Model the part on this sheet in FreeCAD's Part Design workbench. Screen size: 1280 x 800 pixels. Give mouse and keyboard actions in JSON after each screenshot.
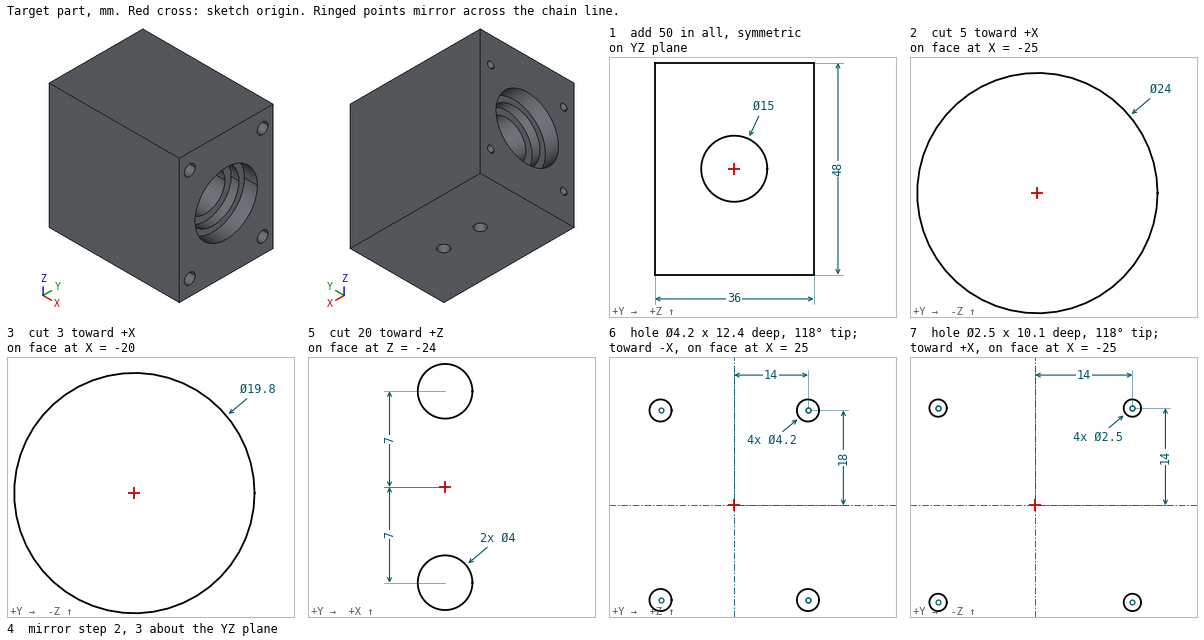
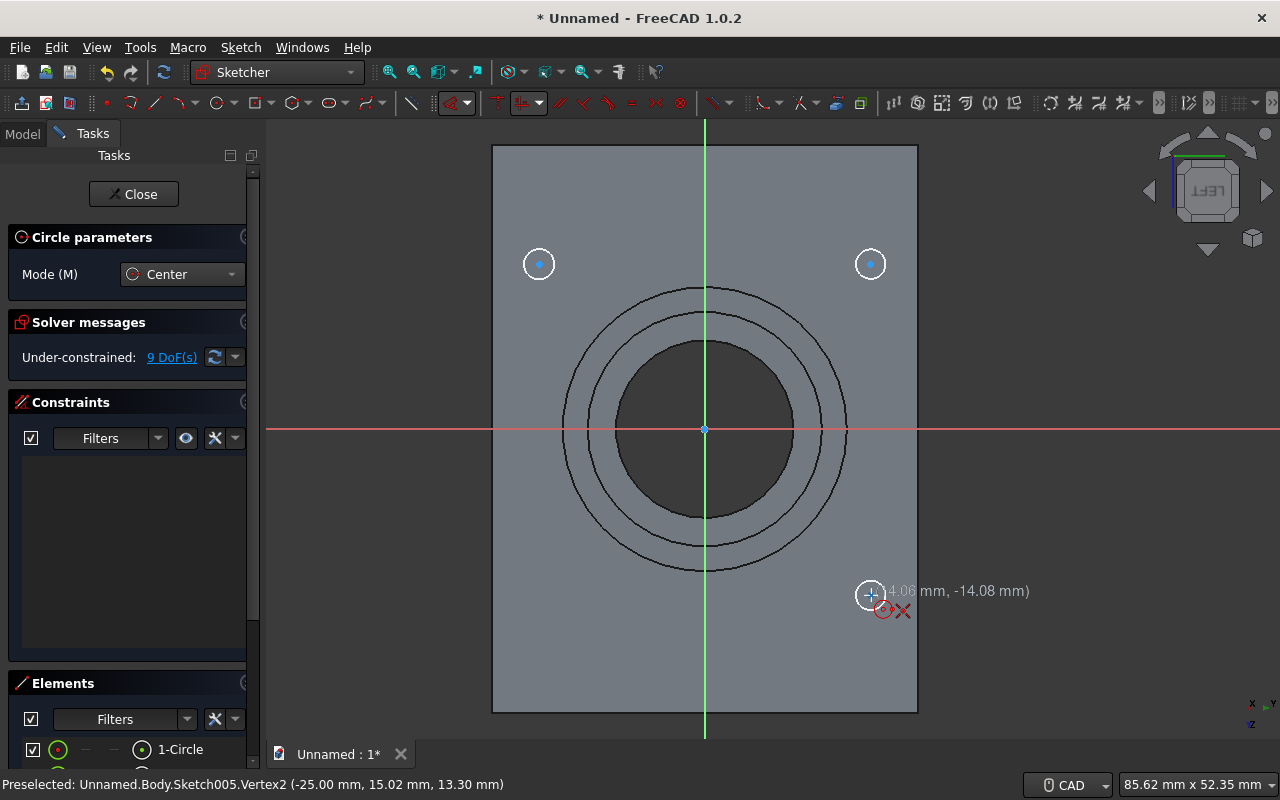
{"action": "scroll", "coordinate": [539, 595], "scroll_direction": "up", "scroll_amount": 3}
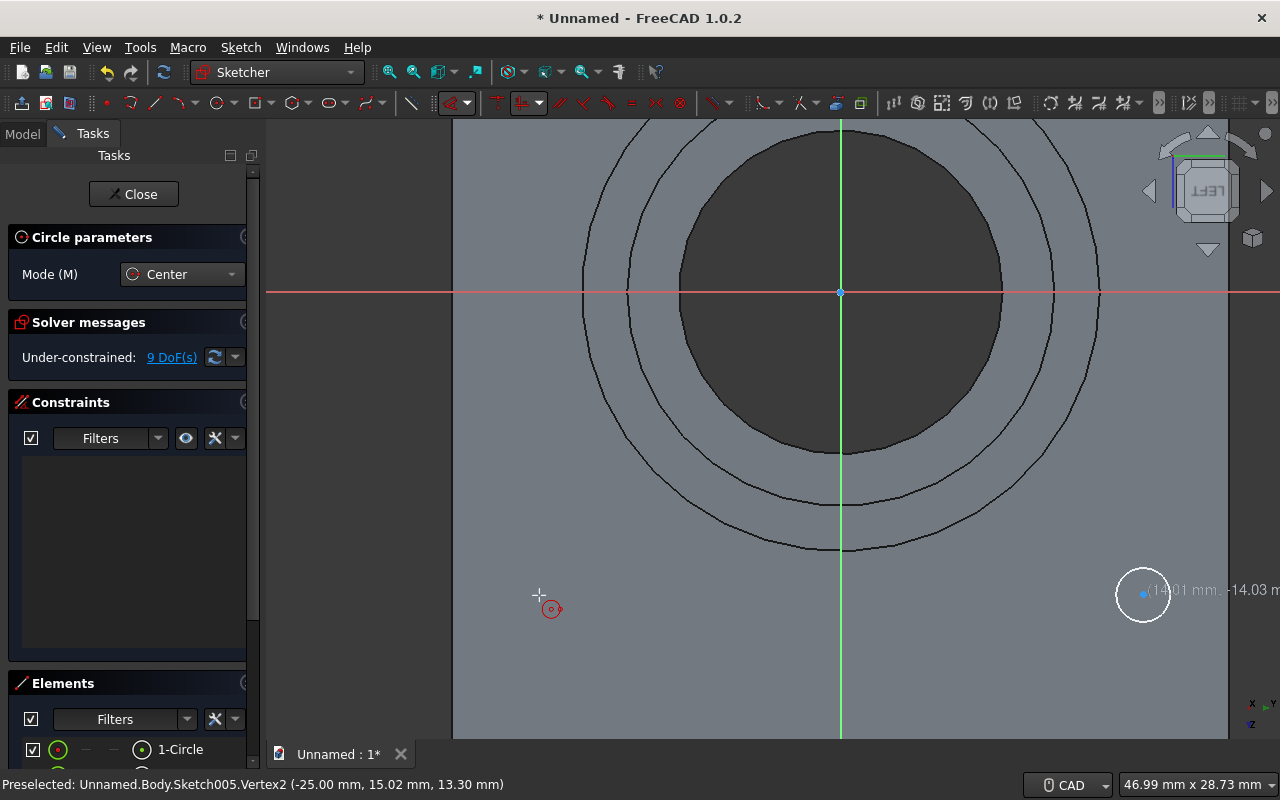
{"action": "left_click", "coordinate": [539, 594]}
{"action": "left_click", "coordinate": [558, 575]}
{"action": "key", "text": "Escape"}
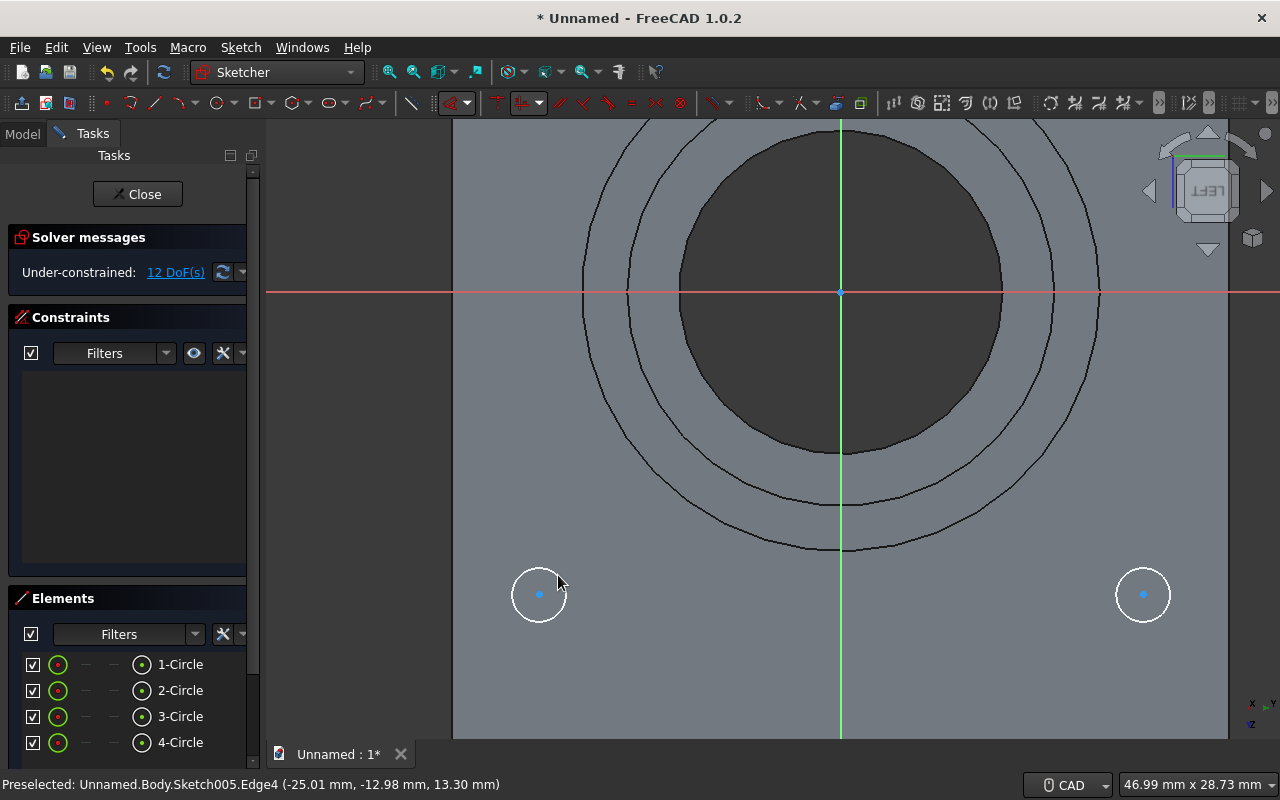
{"action": "scroll", "coordinate": [539, 595], "scroll_direction": "down", "scroll_amount": 3}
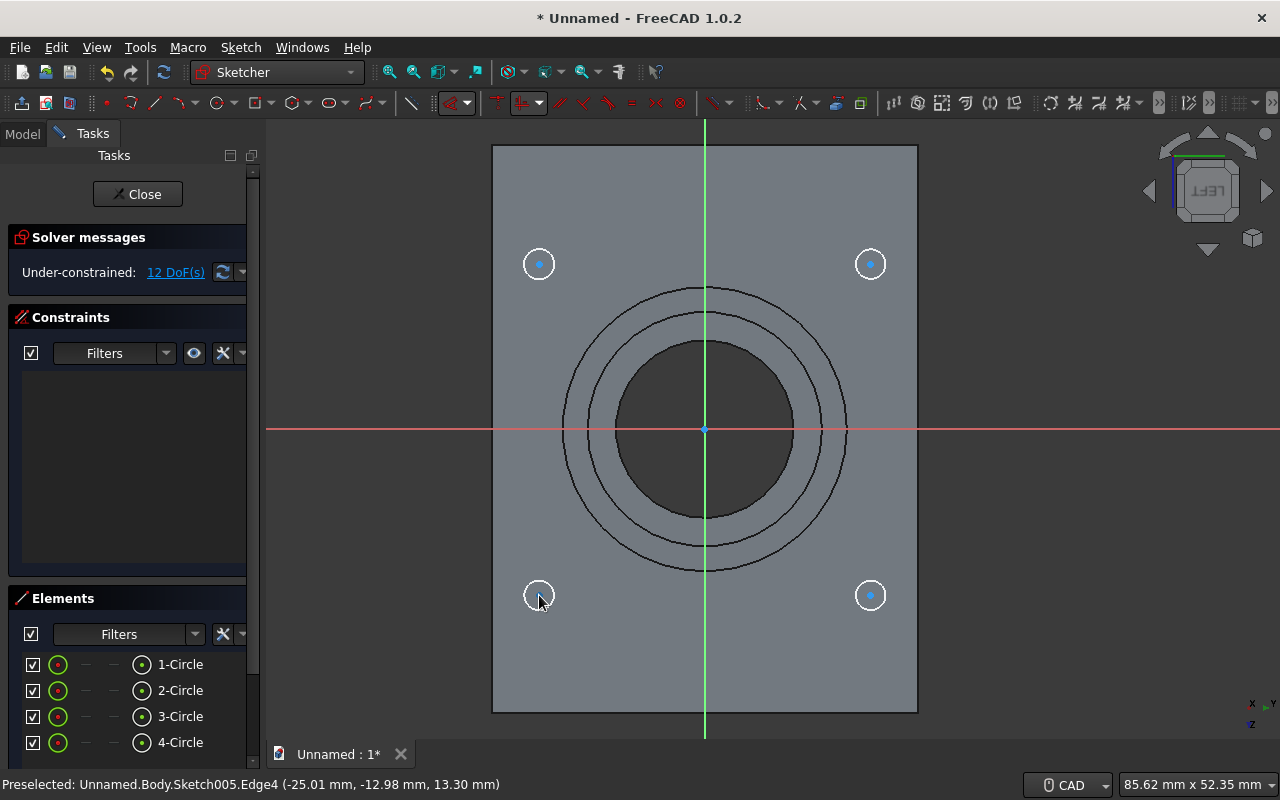
{"action": "left_click", "coordinate": [881, 254]}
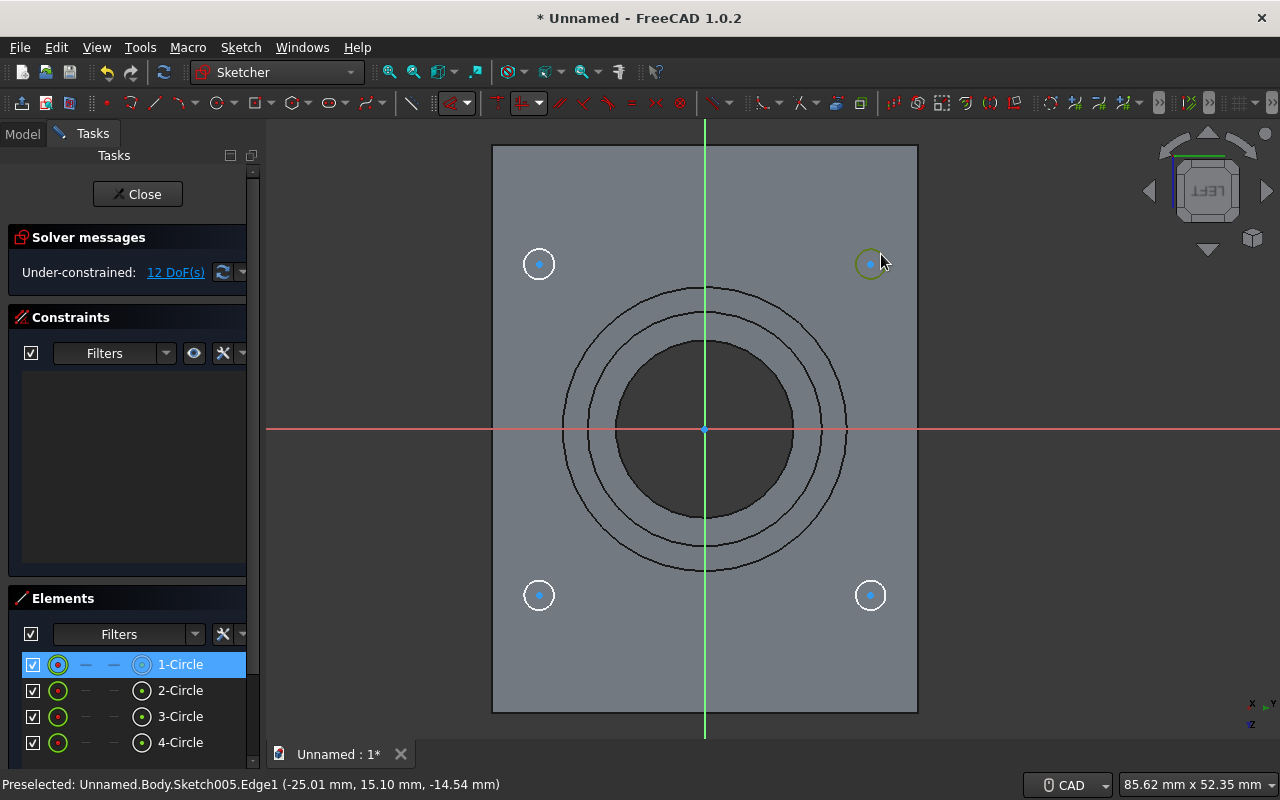
{"action": "left_click", "coordinate": [550, 253]}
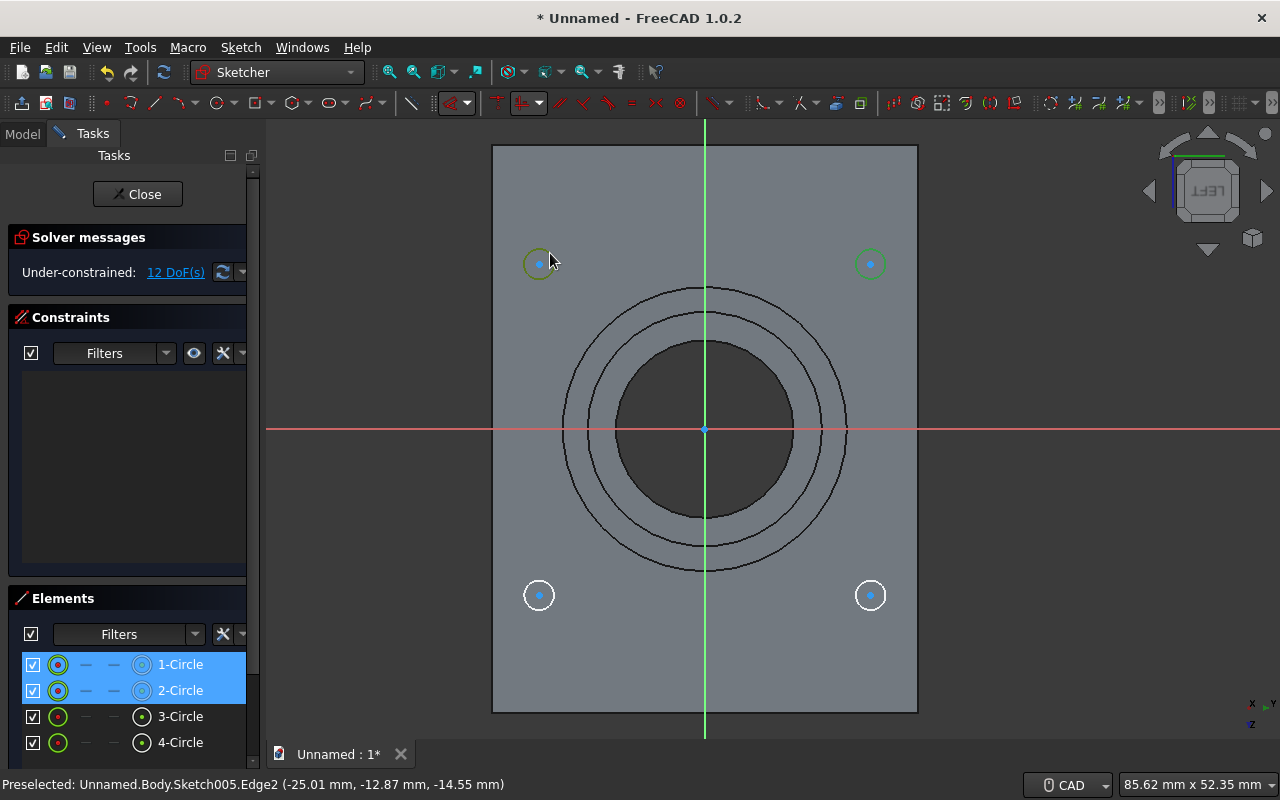
{"action": "left_click", "coordinate": [881, 585]}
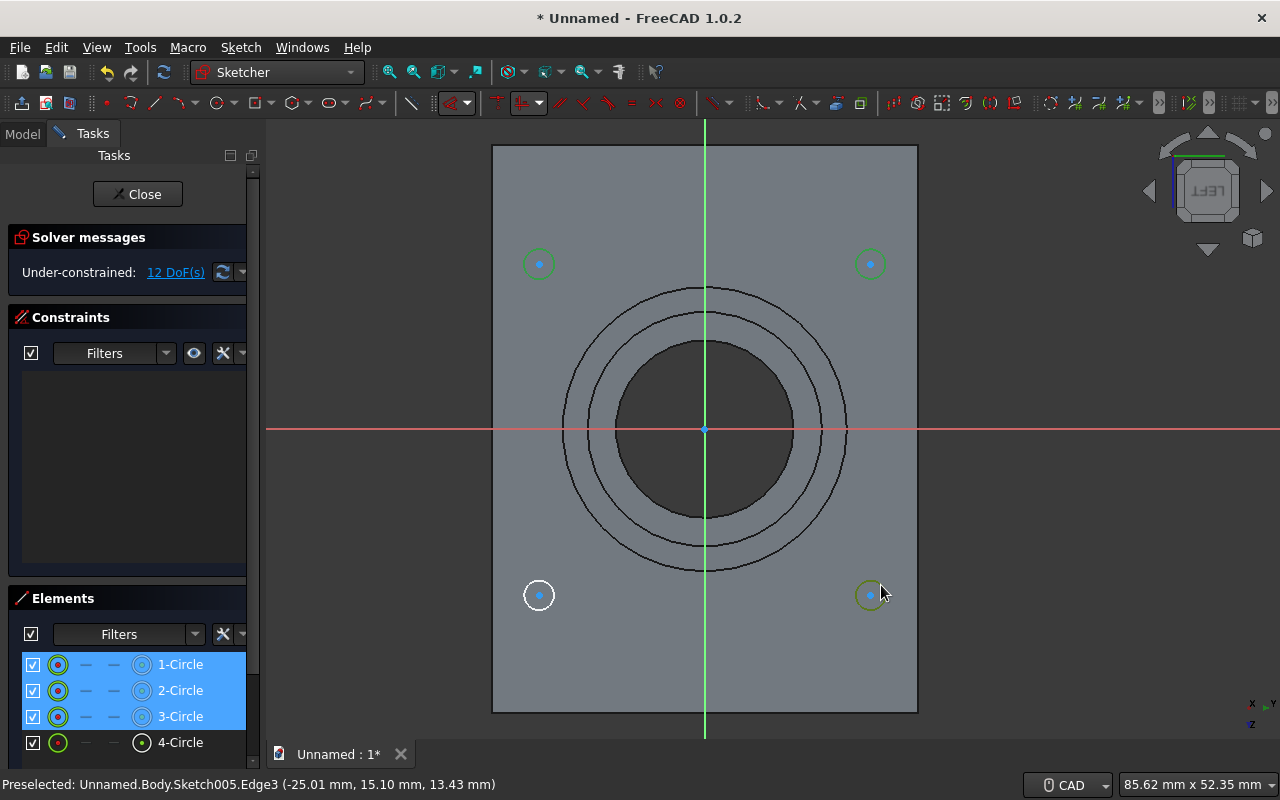
{"action": "left_click", "coordinate": [550, 585]}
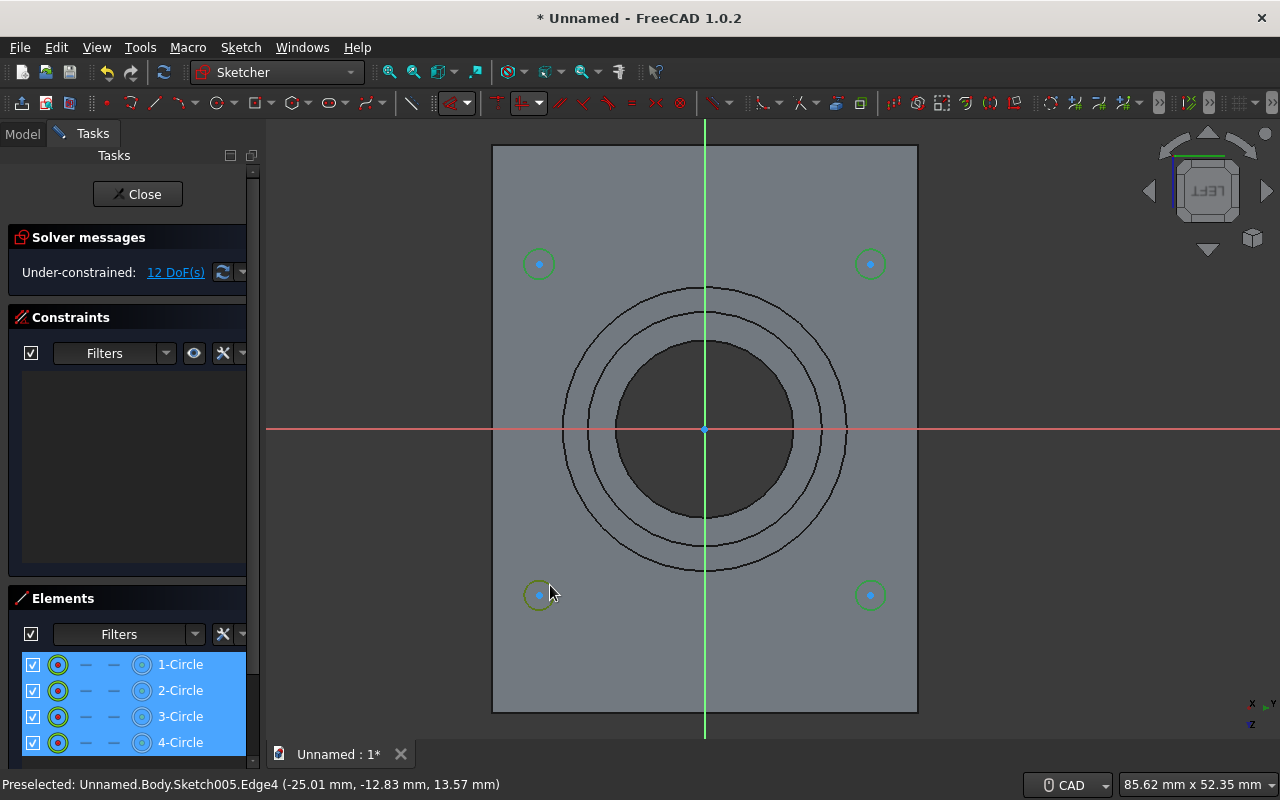
{"action": "left_click", "coordinate": [632, 104]}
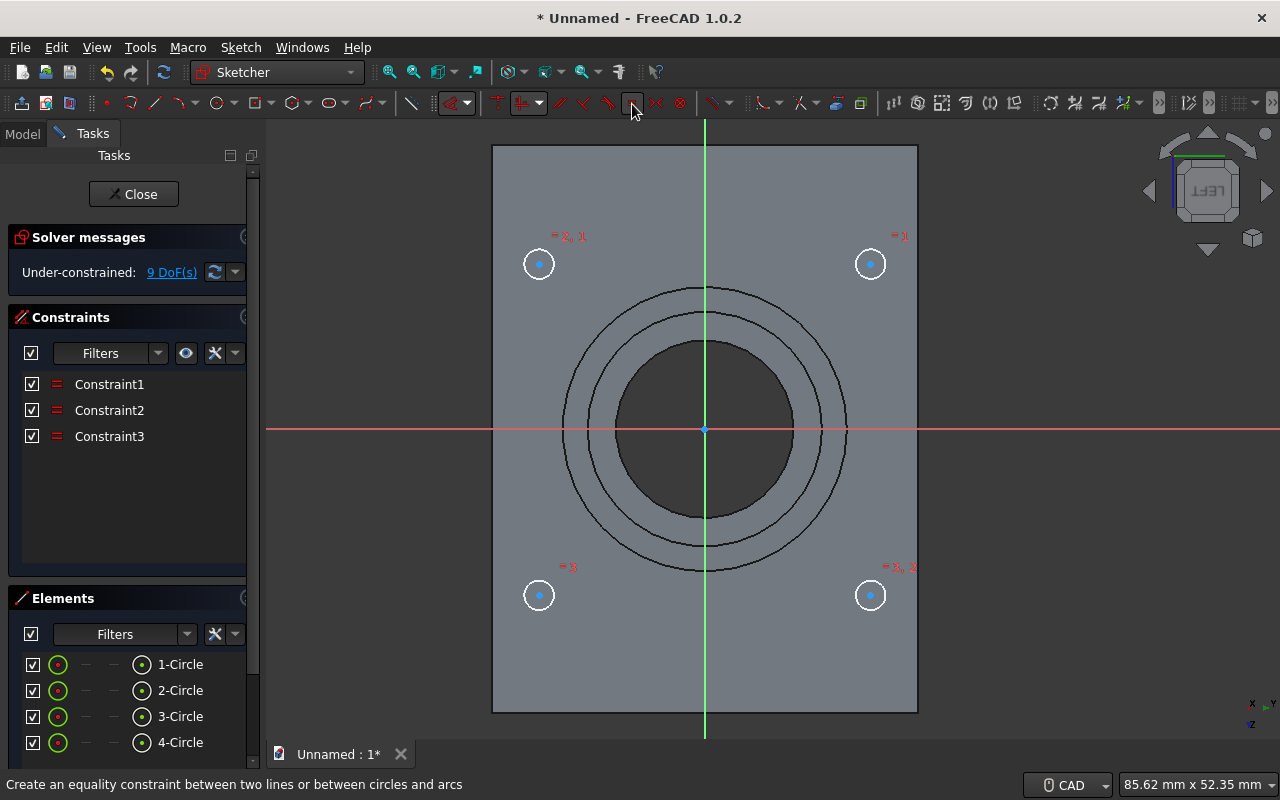
{"action": "left_click", "coordinate": [871, 264]}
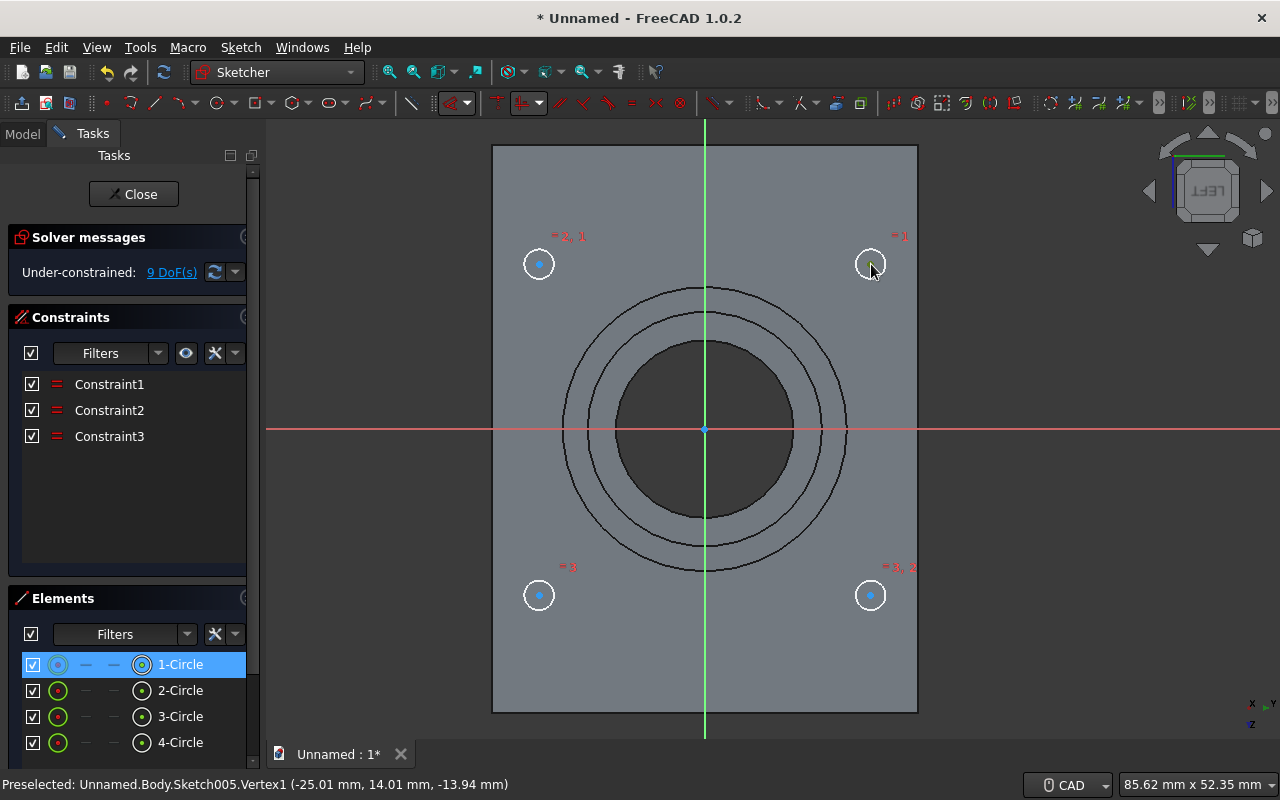
{"action": "left_click", "coordinate": [539, 264]}